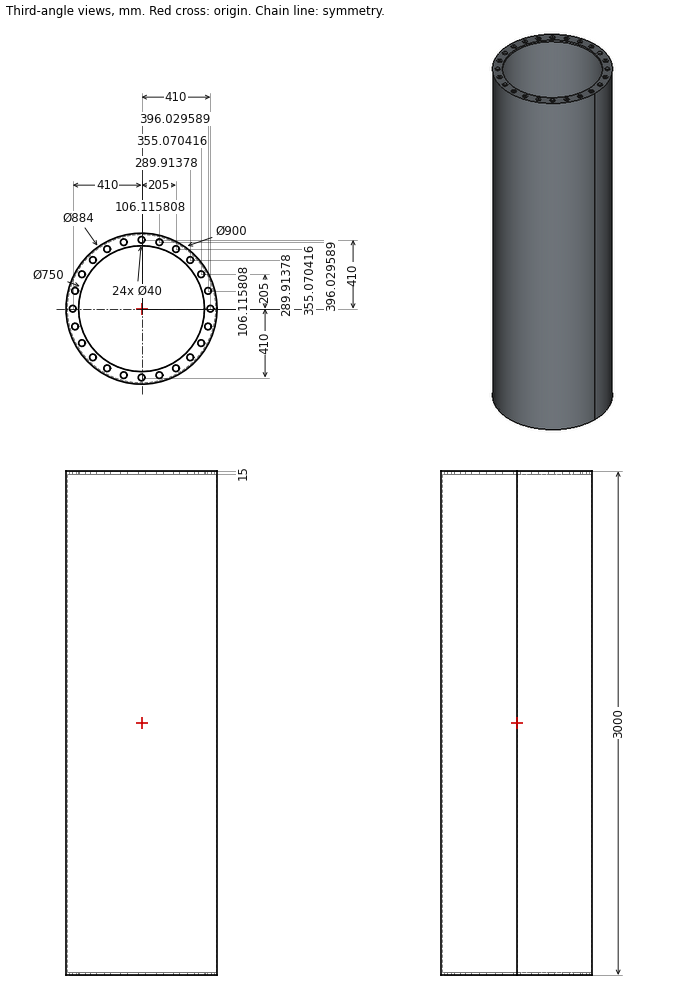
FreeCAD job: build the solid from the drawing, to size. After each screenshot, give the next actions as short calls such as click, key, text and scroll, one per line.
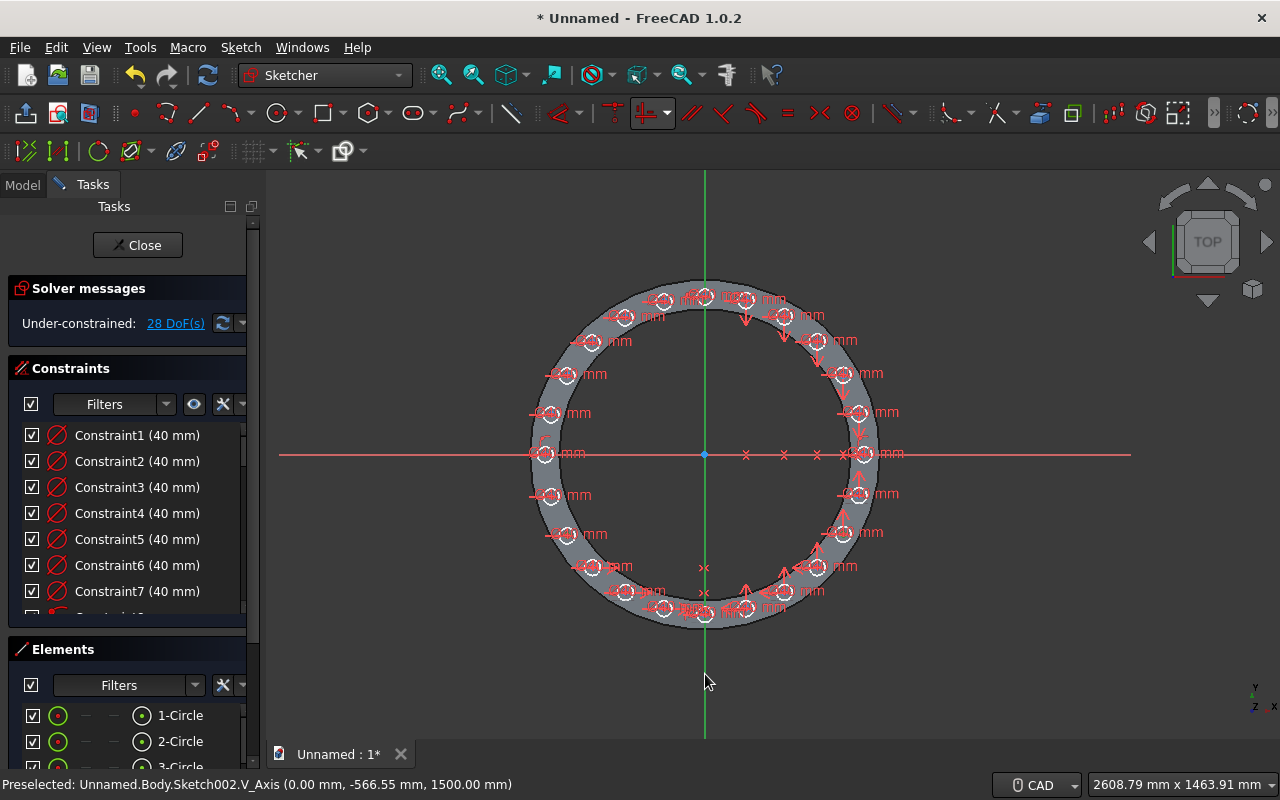
click(820, 114)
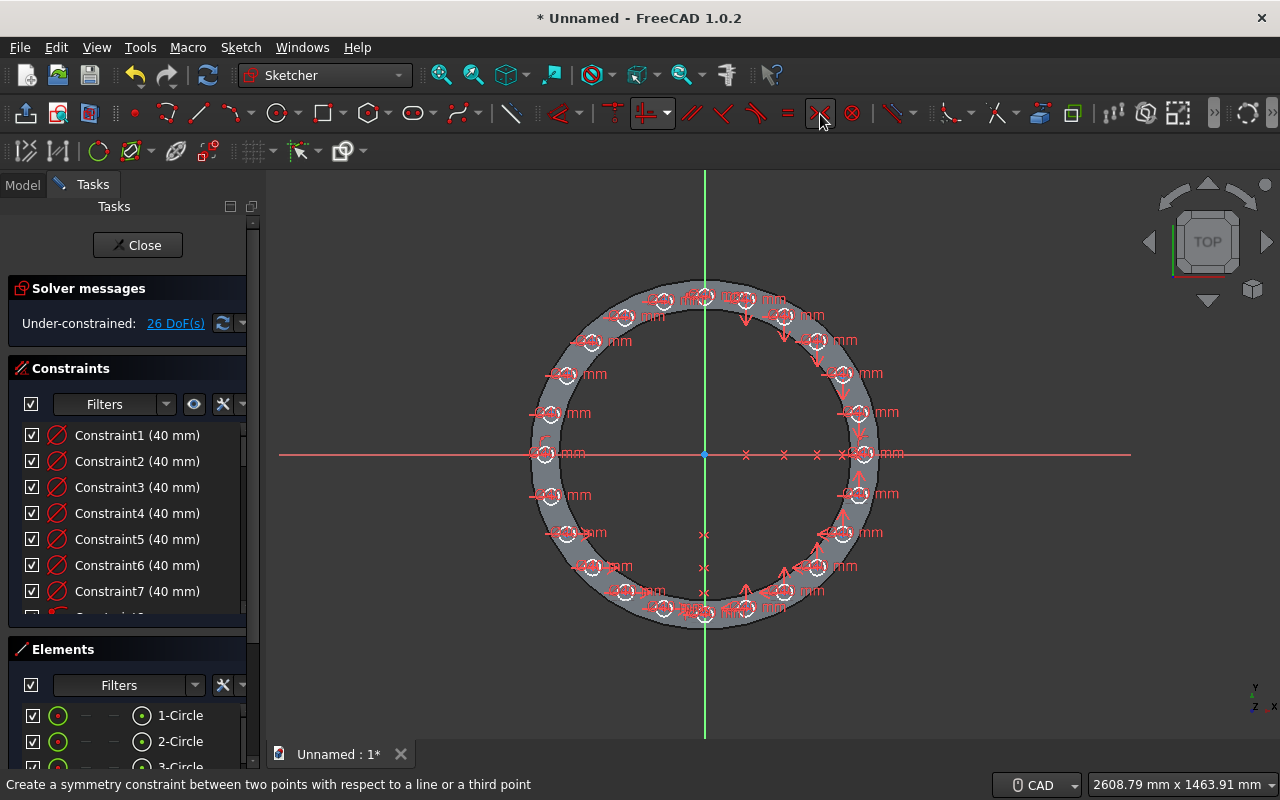
click(859, 496)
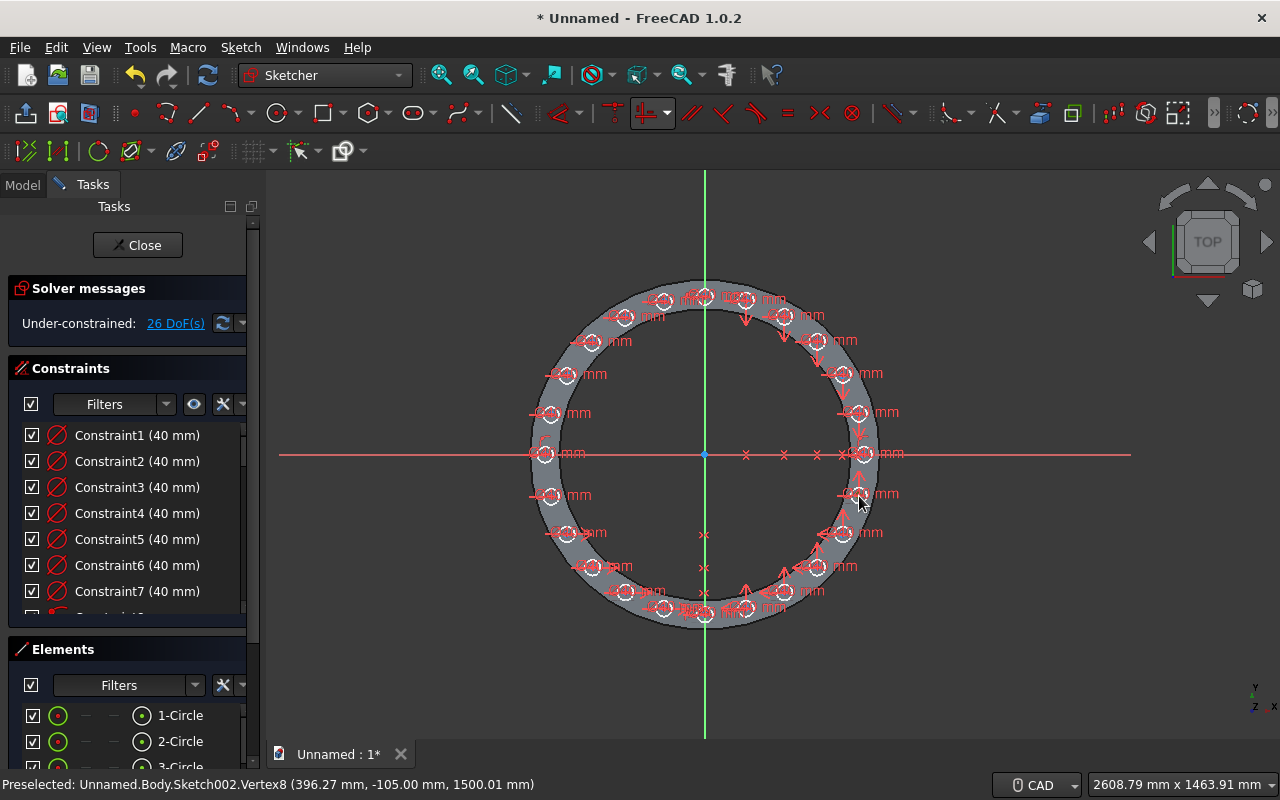
click(551, 497)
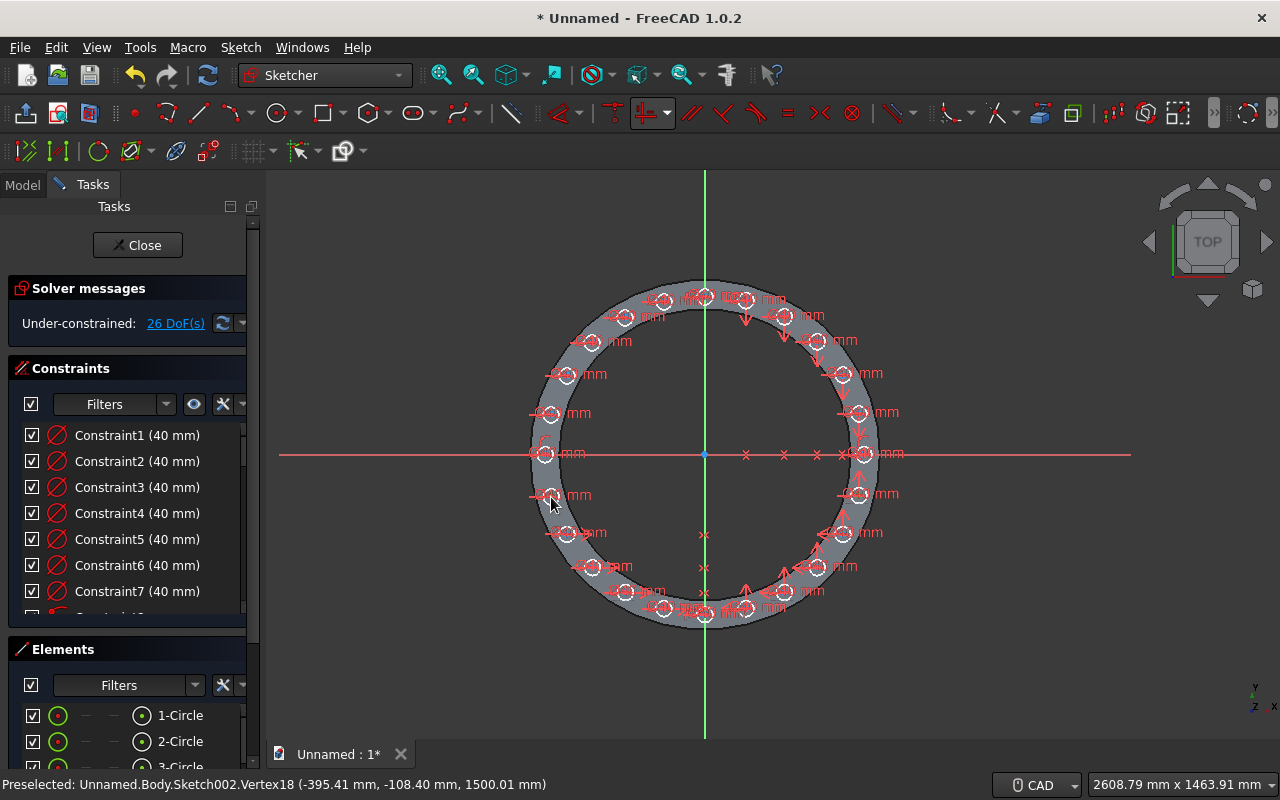
click(705, 674)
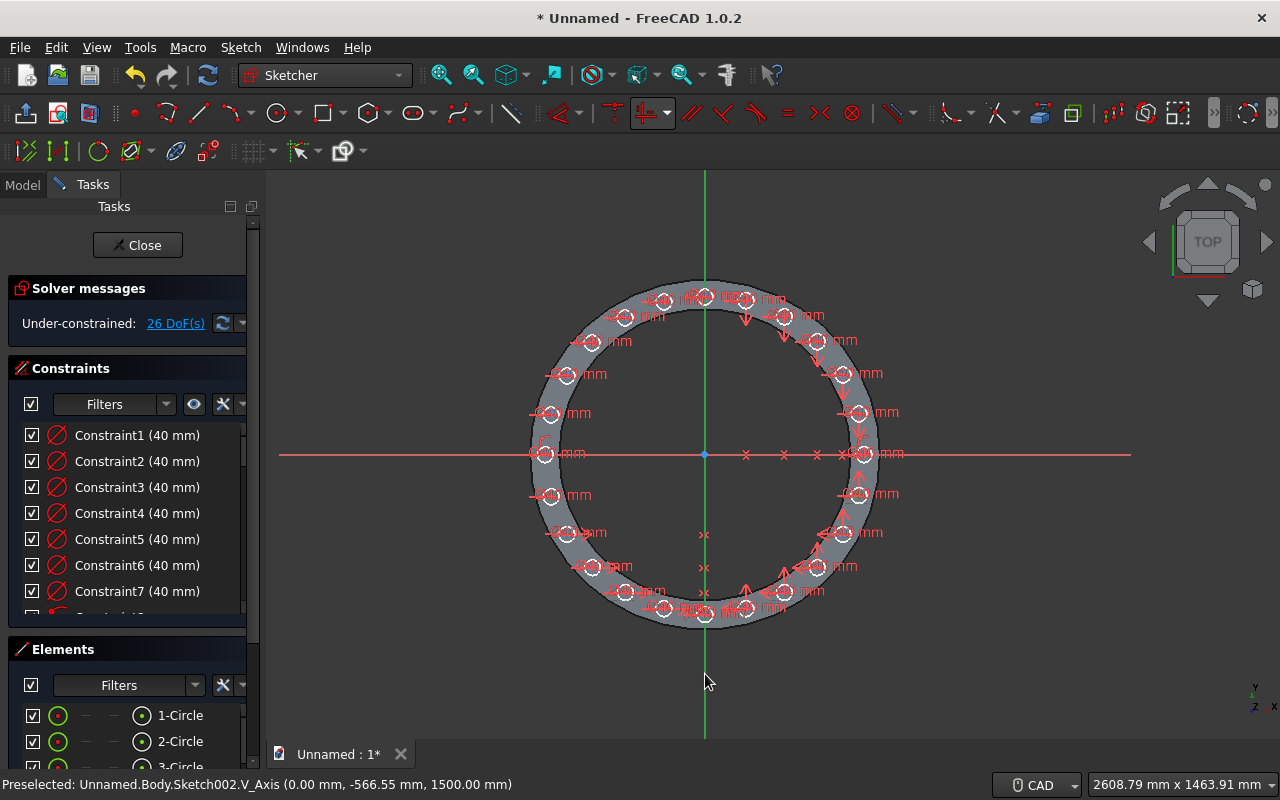
click(820, 114)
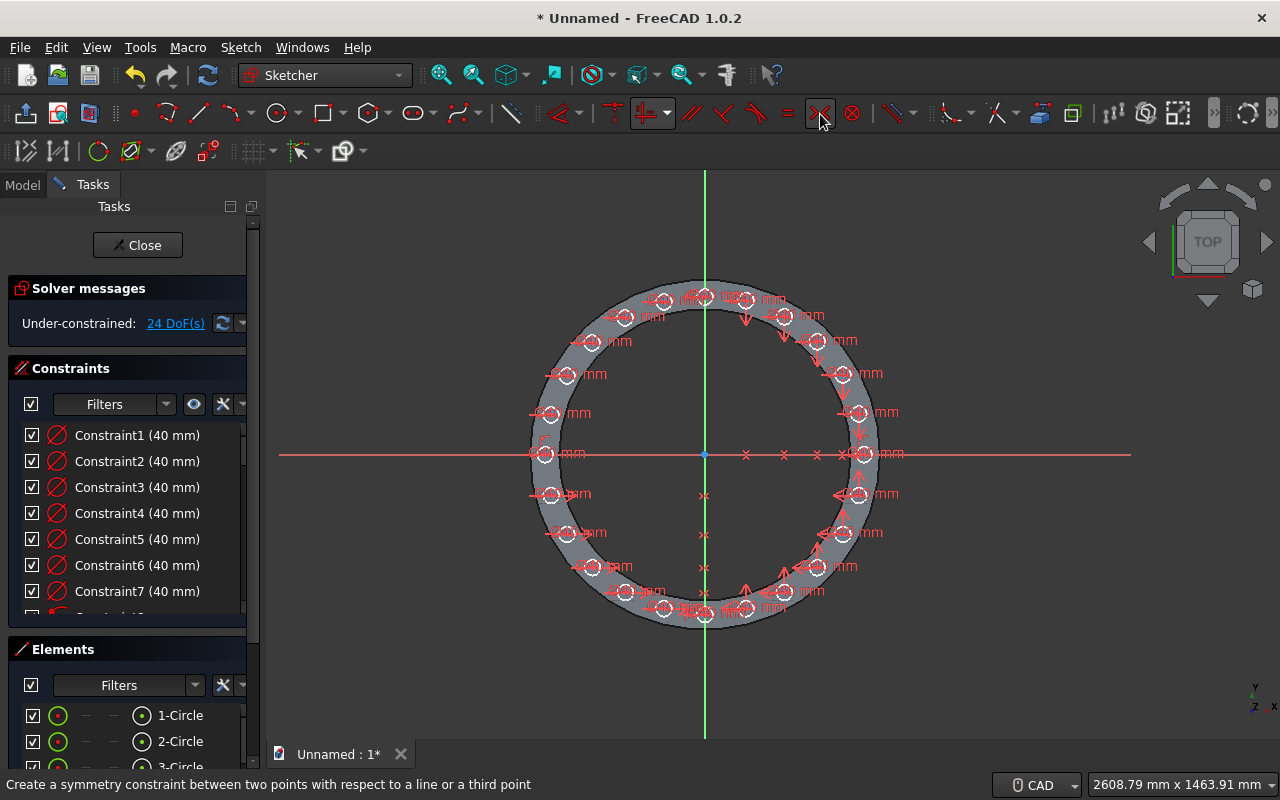
click(859, 414)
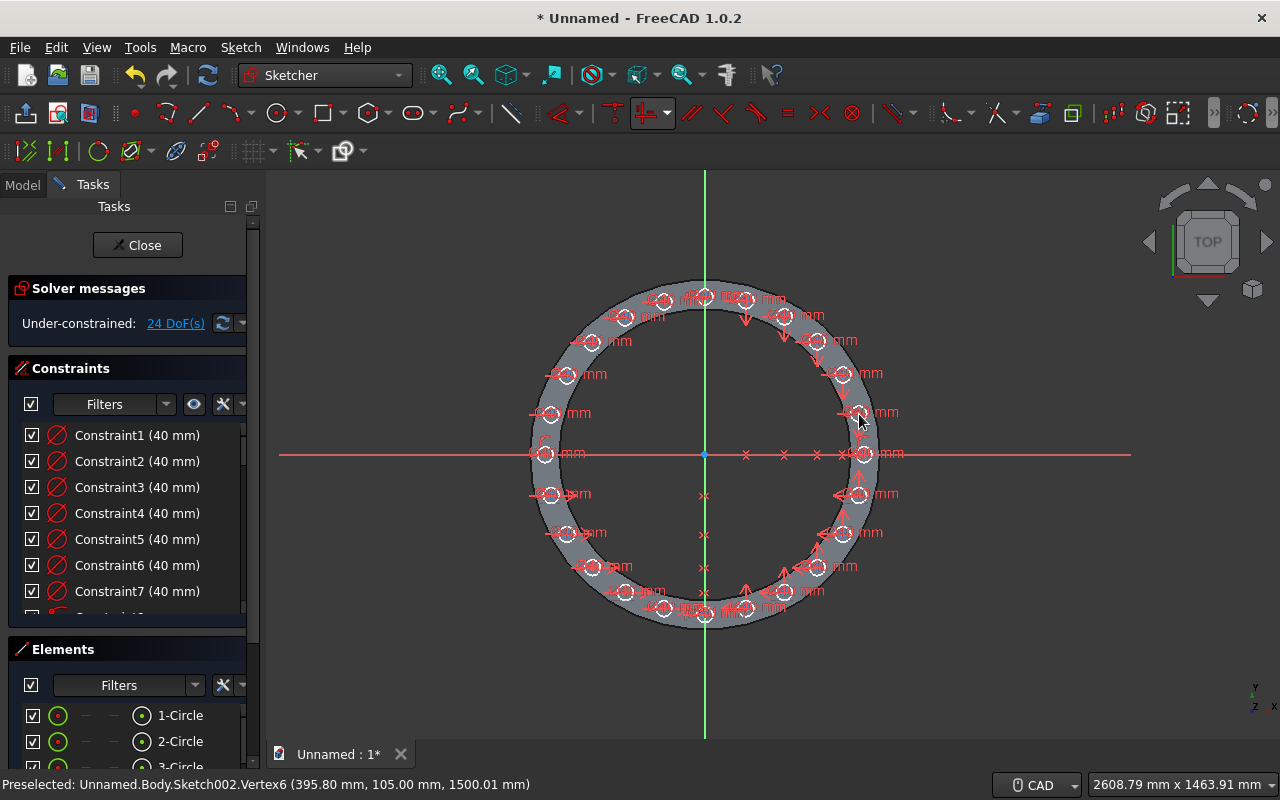
click(551, 415)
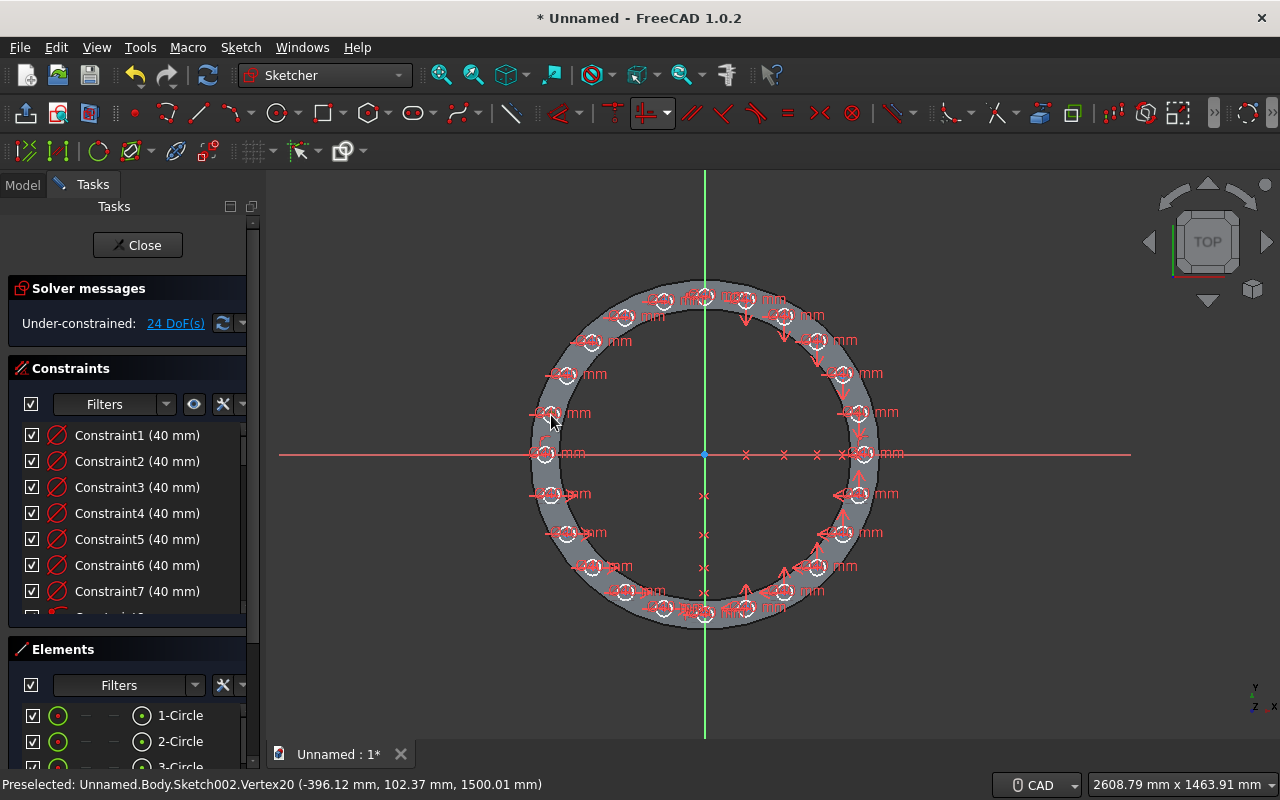
click(705, 674)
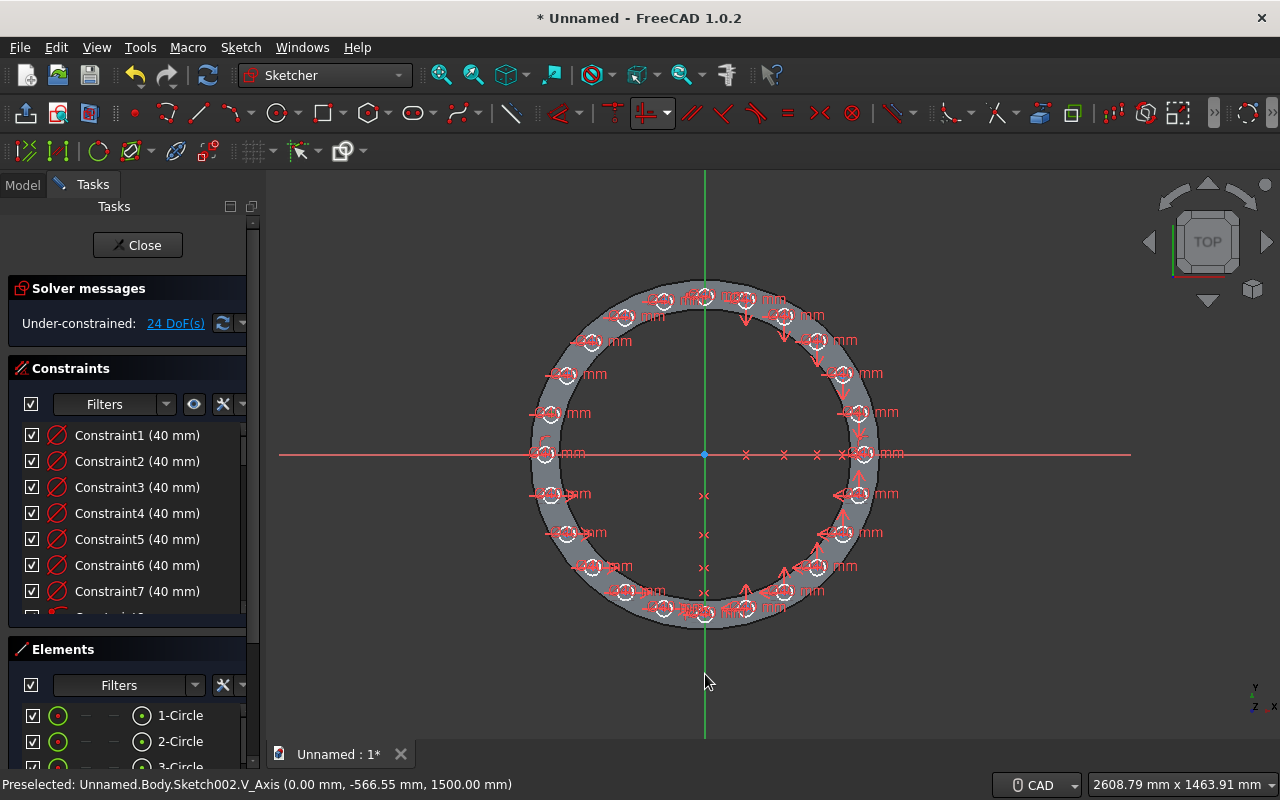
click(820, 114)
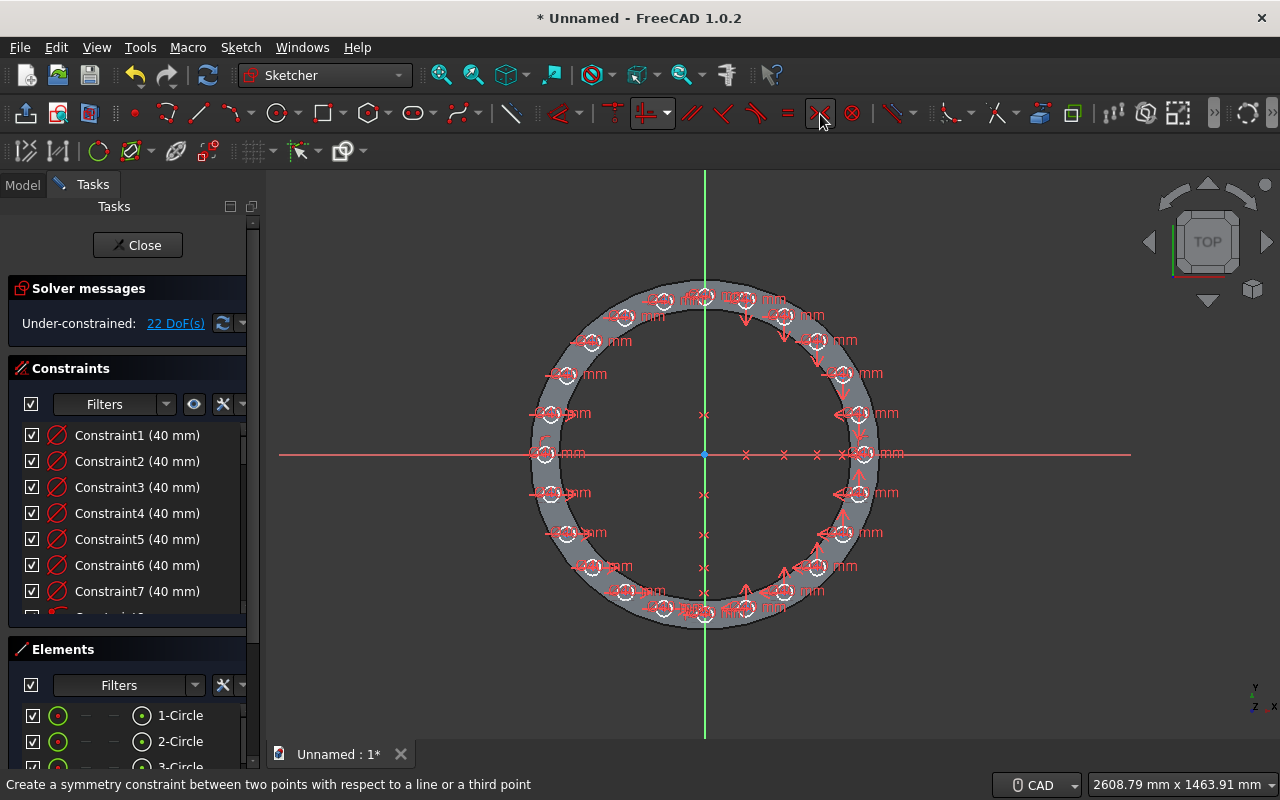
click(843, 375)